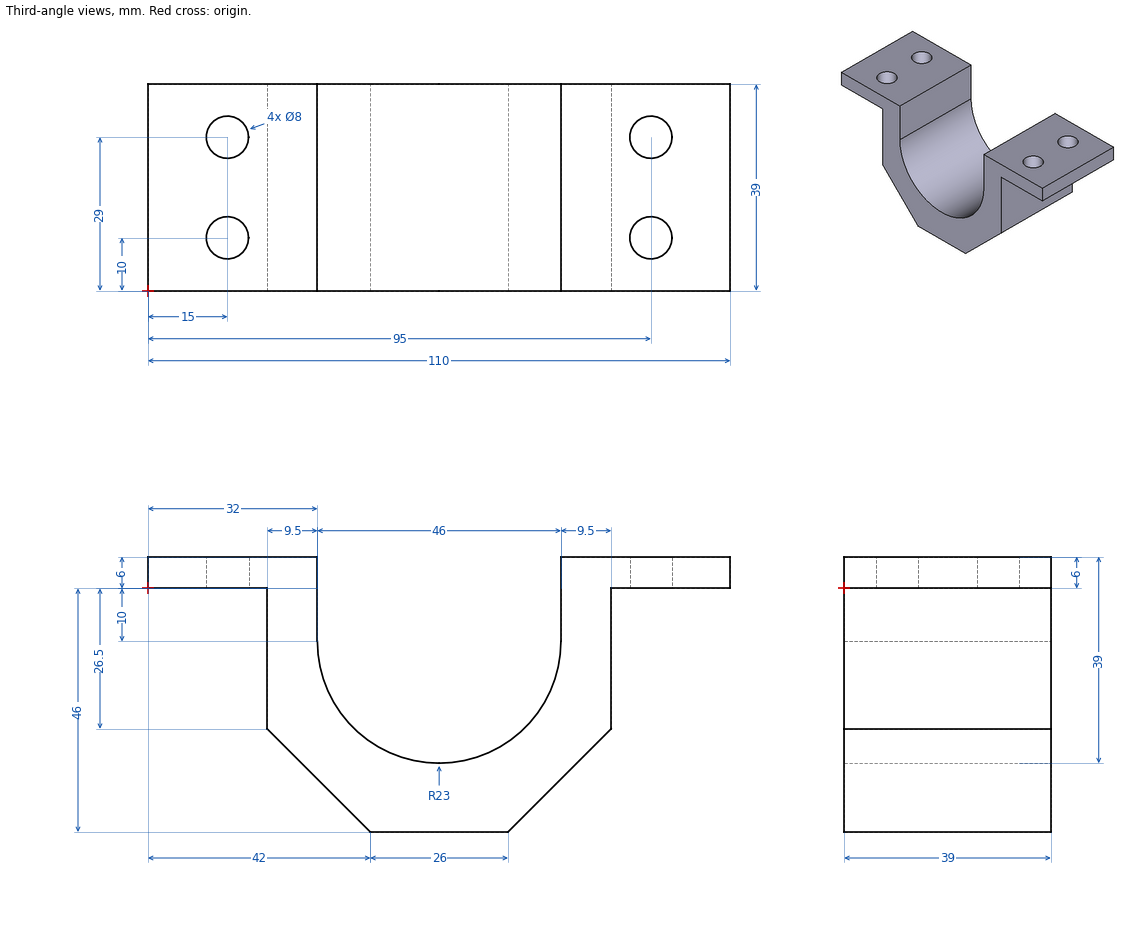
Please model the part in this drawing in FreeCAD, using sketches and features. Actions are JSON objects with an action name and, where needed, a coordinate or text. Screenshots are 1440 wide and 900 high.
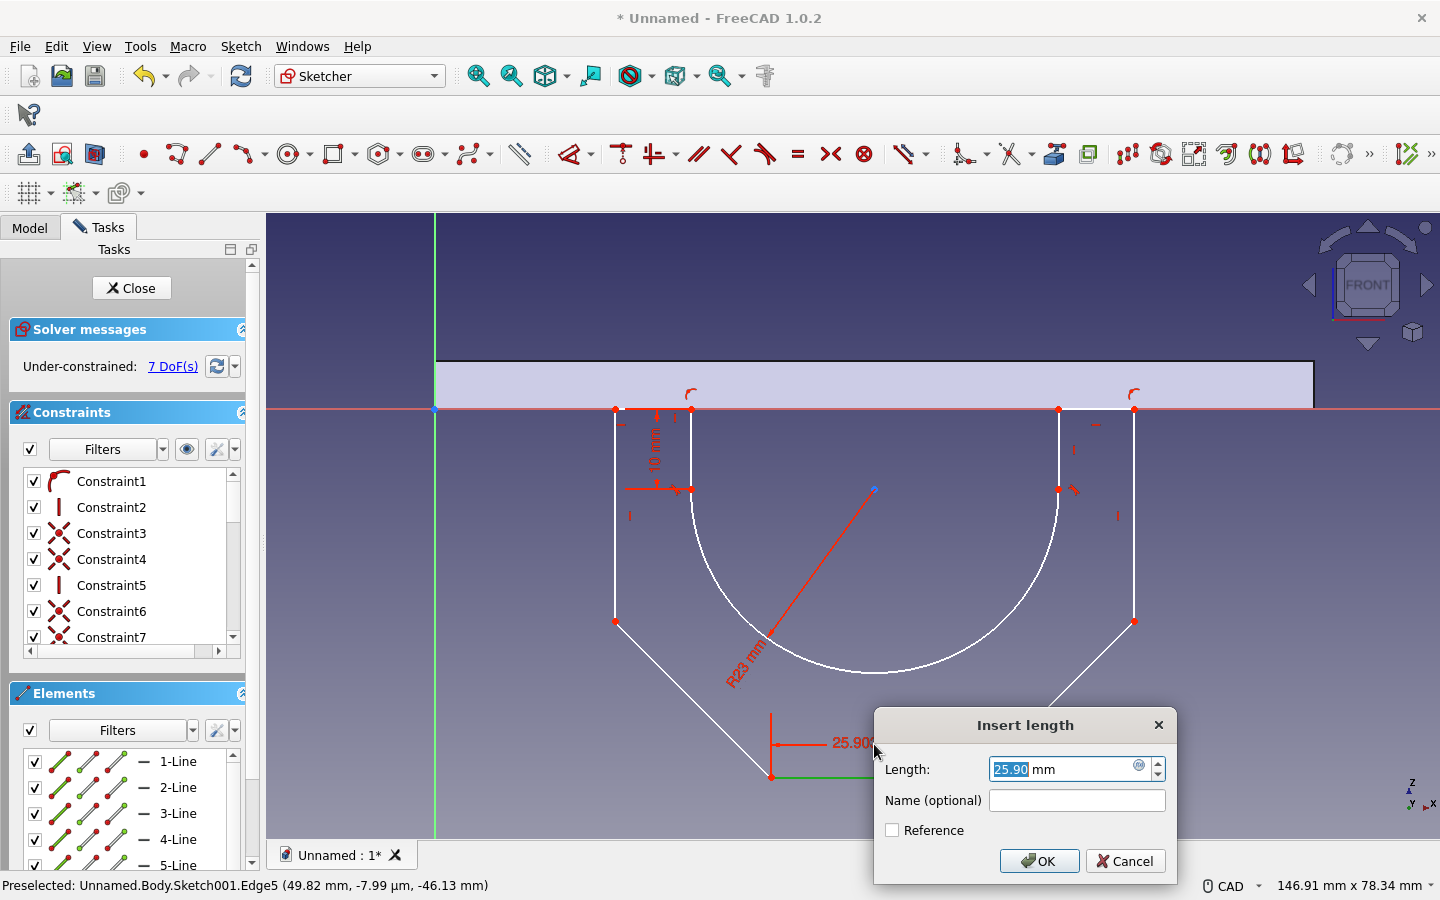
{"action": "type", "text": "26"}
{"action": "key", "text": "Return"}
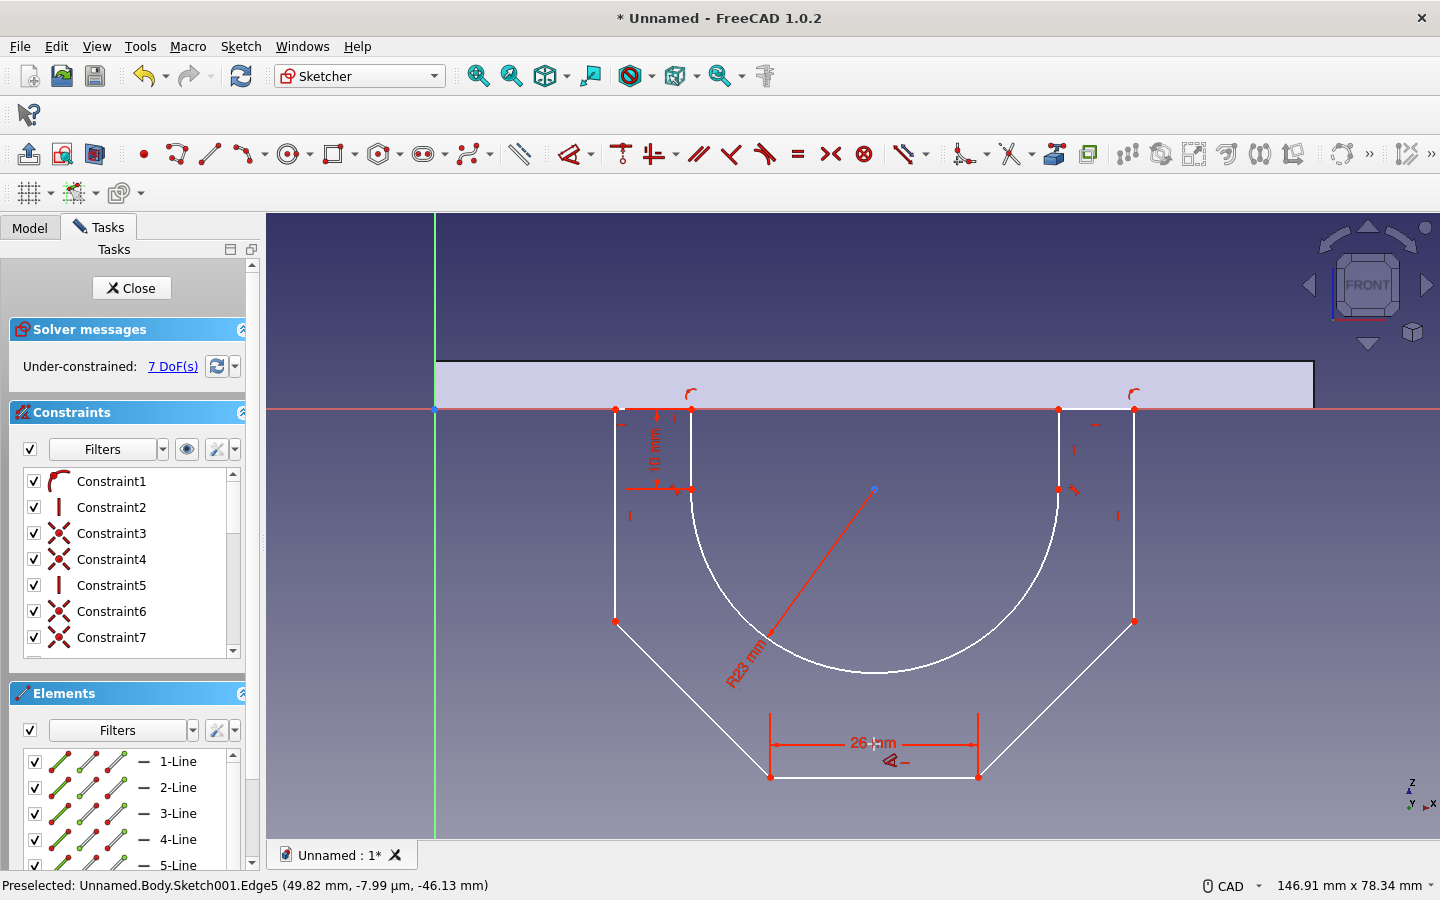
{"action": "left_click", "coordinate": [668, 409]}
{"action": "left_click", "coordinate": [653, 375]}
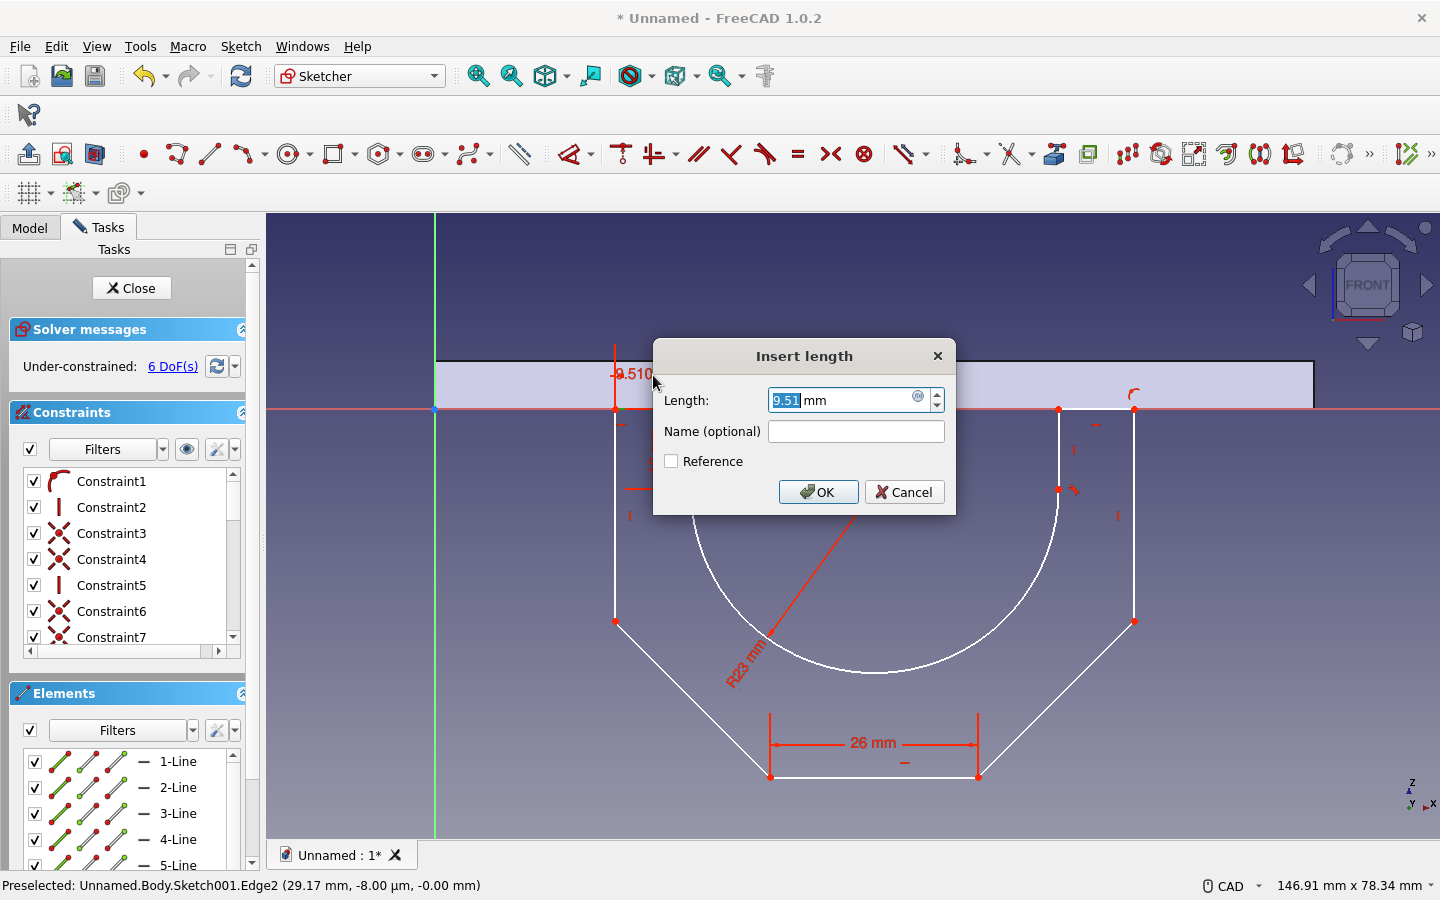
{"action": "type", "text": "9.5"}
{"action": "key", "text": "Return"}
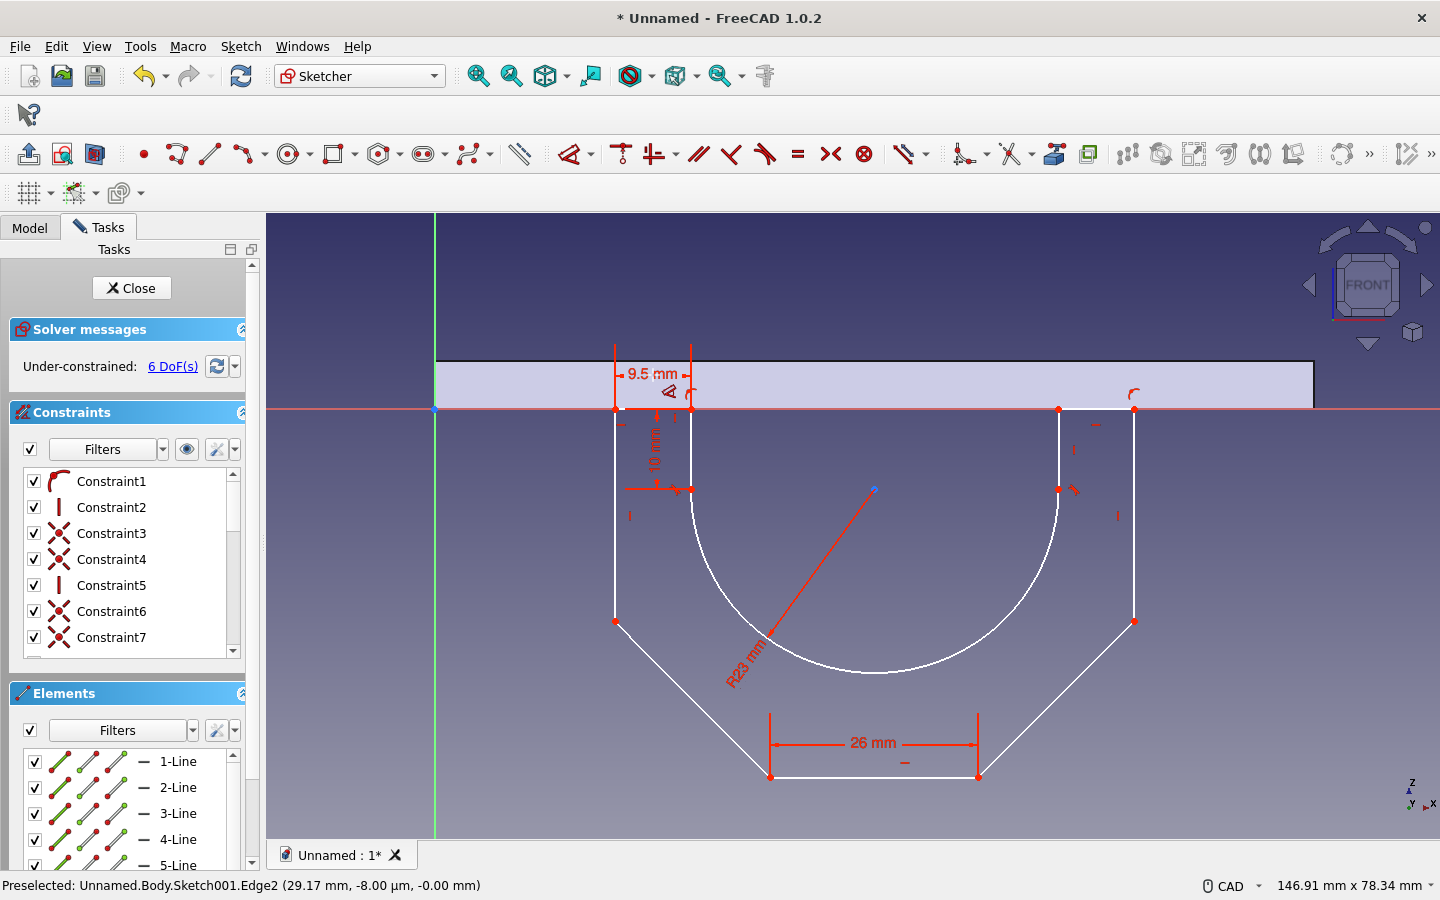
{"action": "left_click", "coordinate": [1111, 409]}
{"action": "left_click", "coordinate": [1096, 375]}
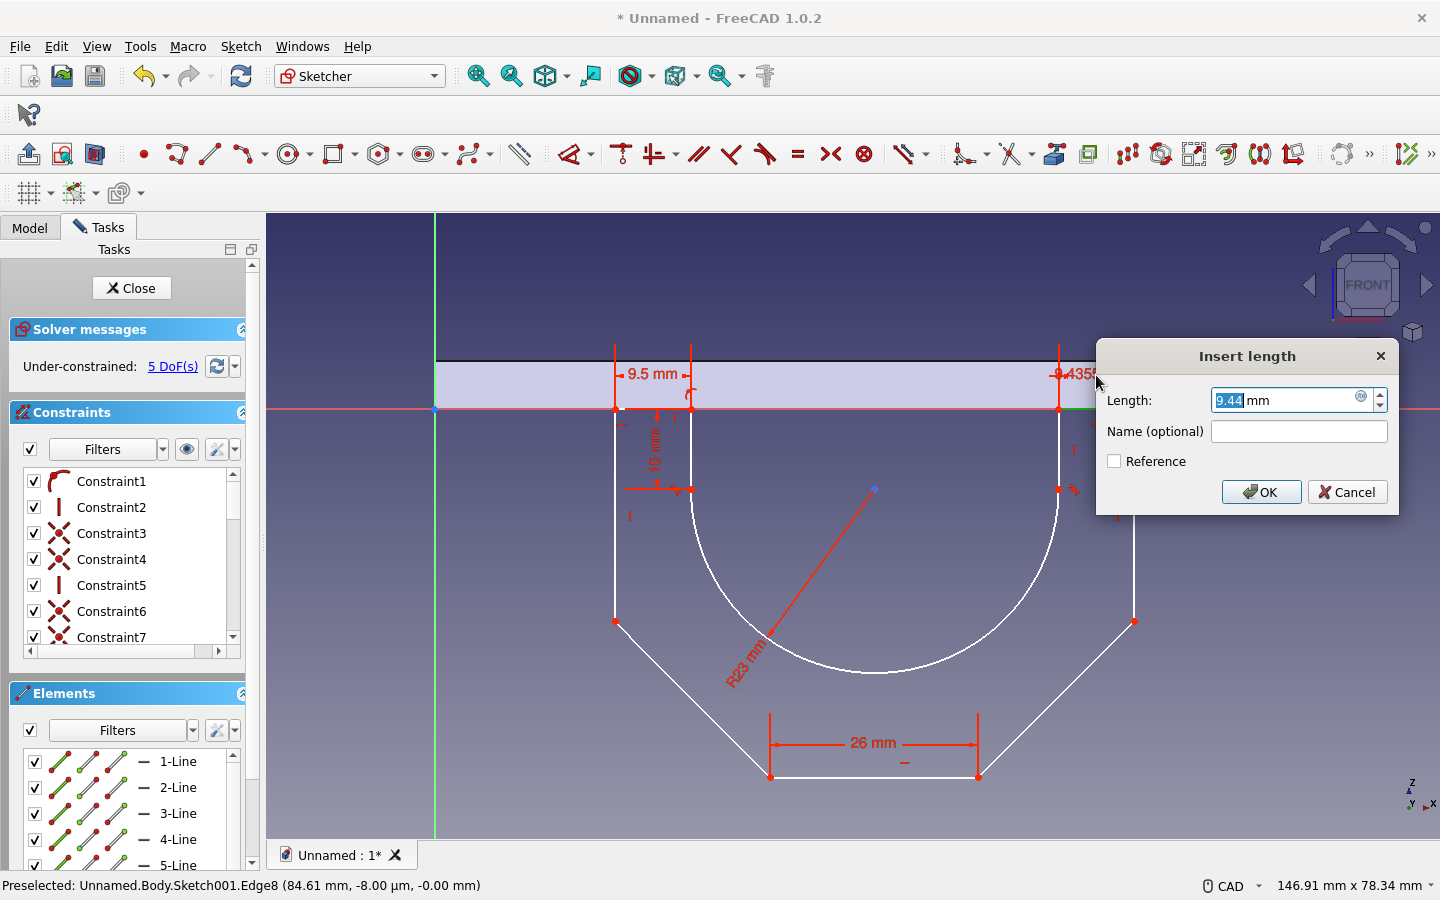
{"action": "type", "text": "9.5"}
{"action": "key", "text": "Return"}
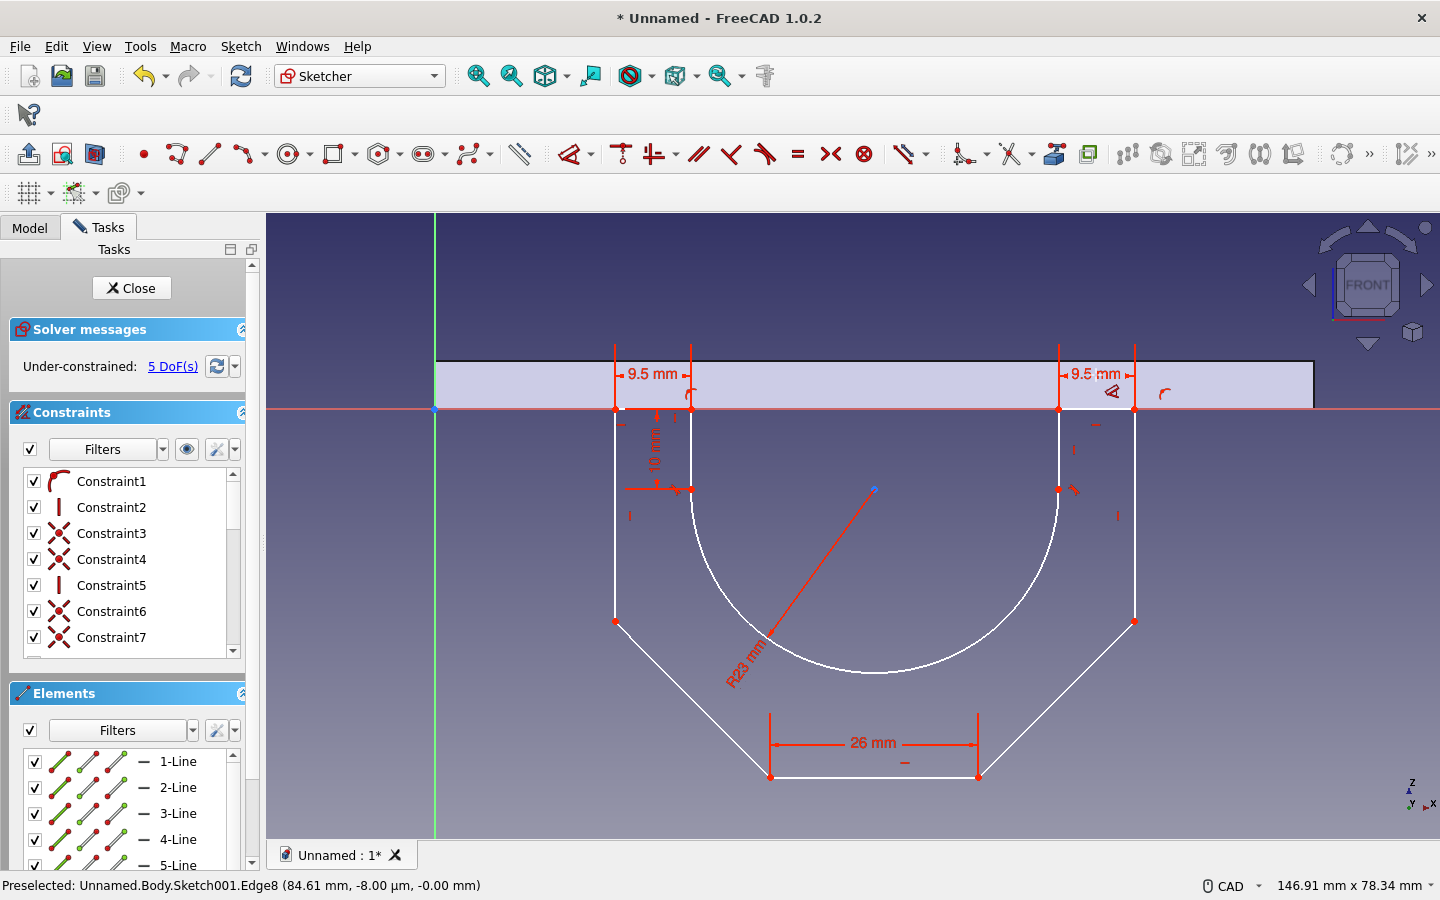
{"action": "left_click", "coordinate": [691, 489]}
{"action": "left_click", "coordinate": [563, 375]}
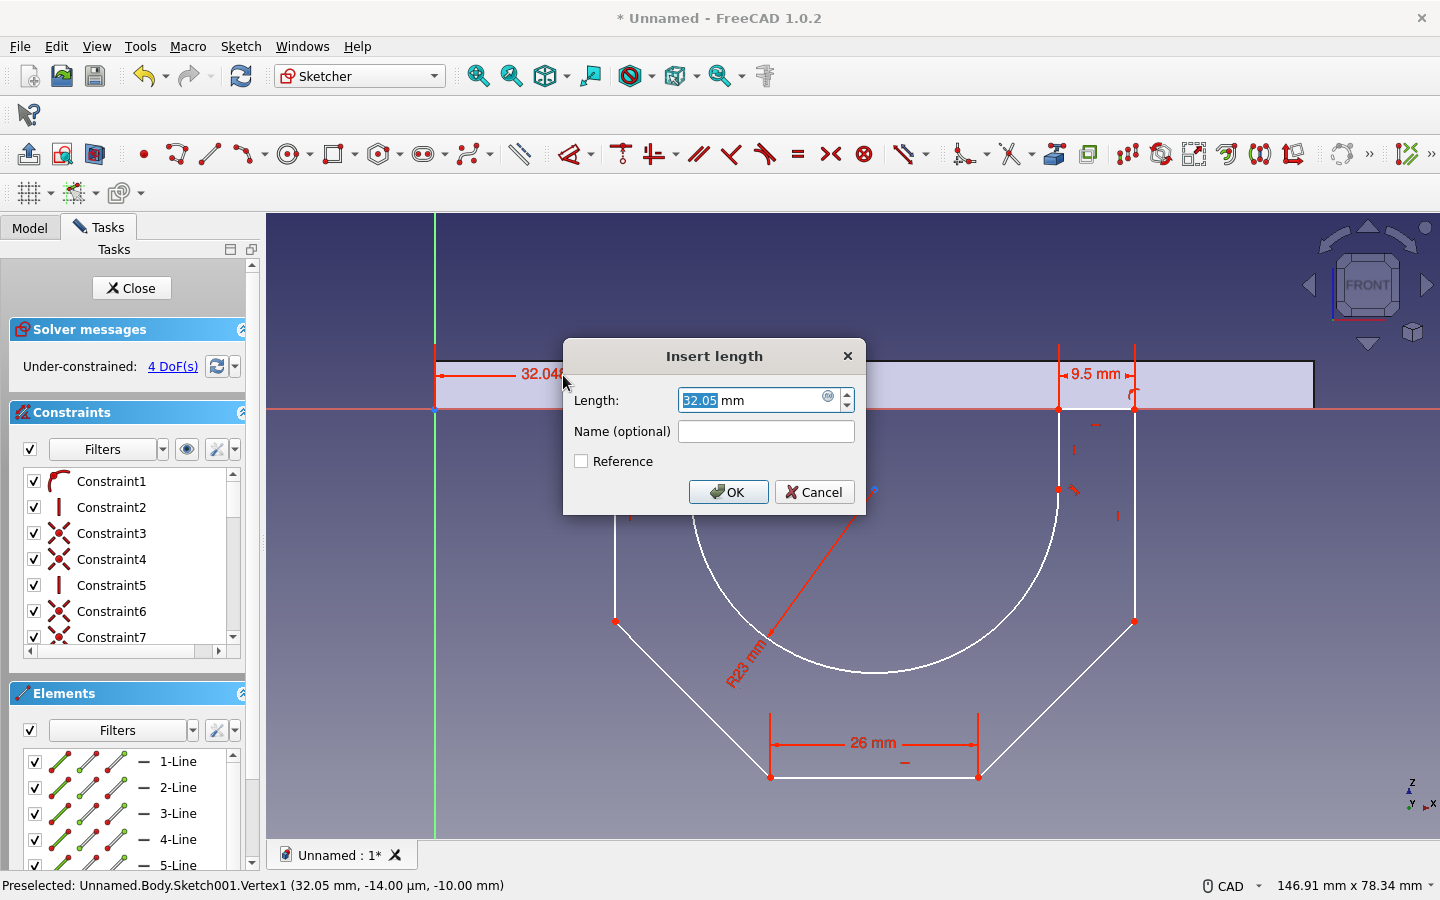
{"action": "type", "text": "32"}
{"action": "key", "text": "Return"}